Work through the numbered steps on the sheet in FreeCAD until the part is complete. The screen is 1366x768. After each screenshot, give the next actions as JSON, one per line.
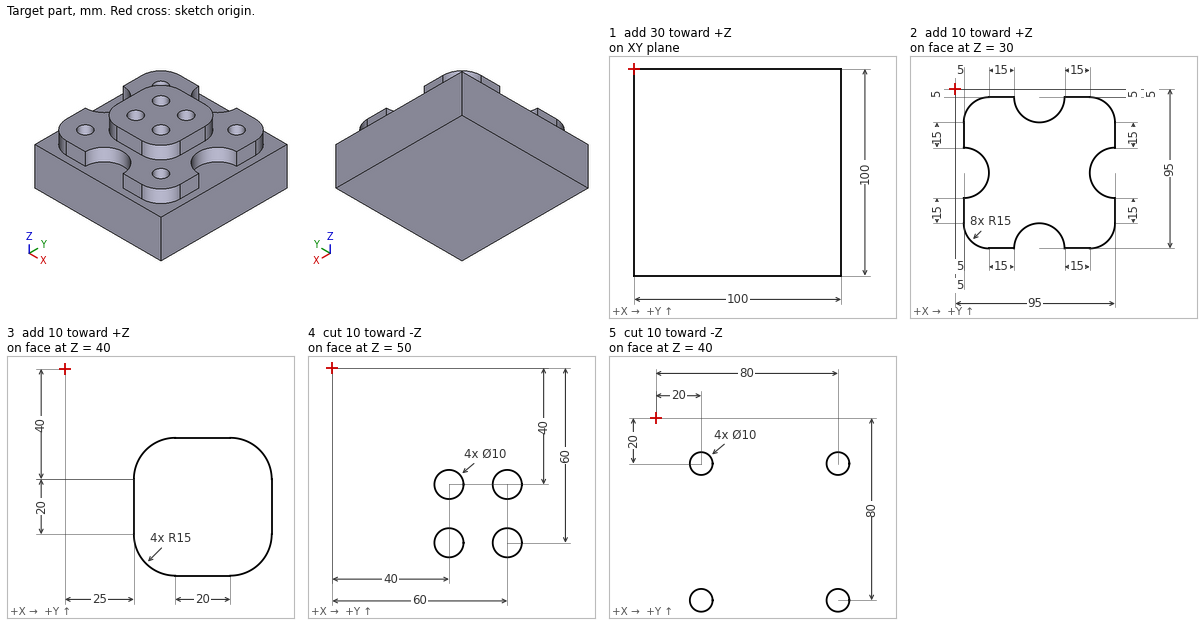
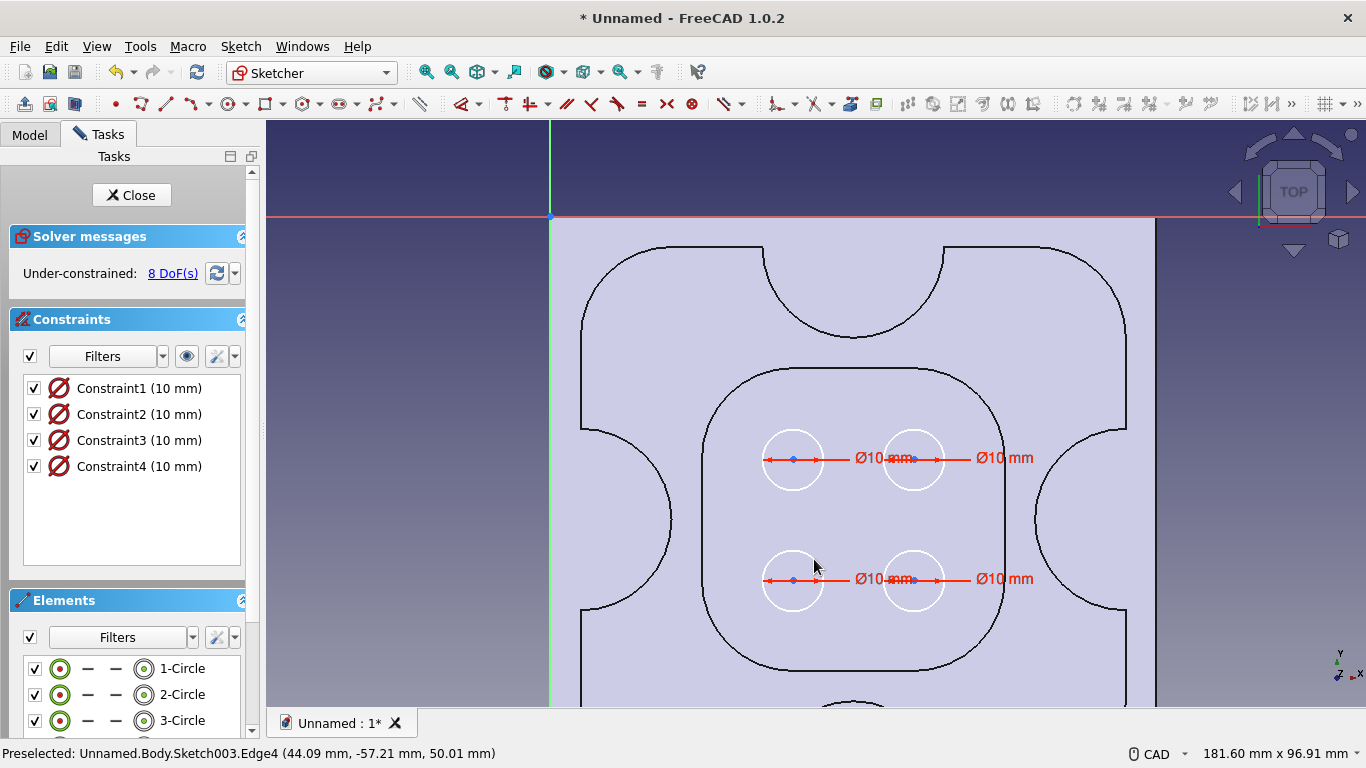
{"action": "left_click", "coordinate": [793, 460]}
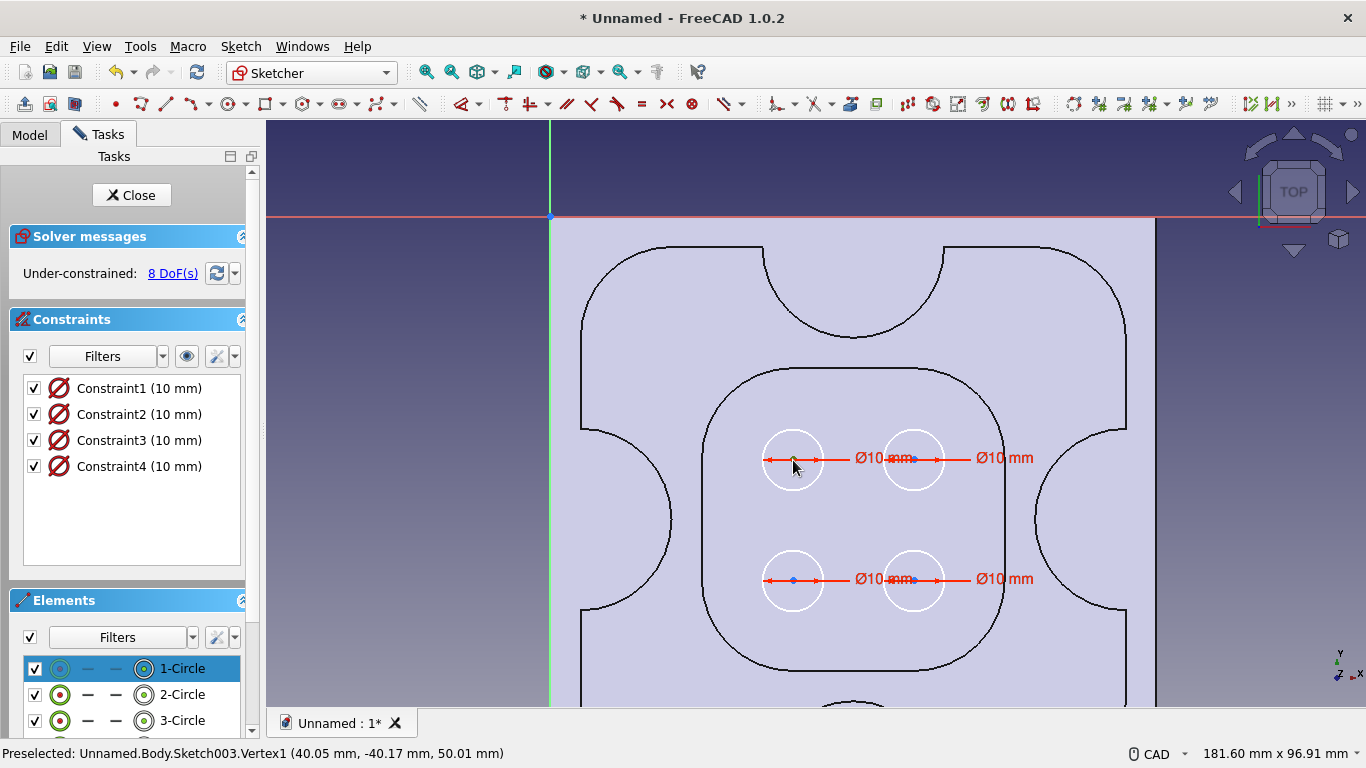
{"action": "left_click", "coordinate": [914, 460]}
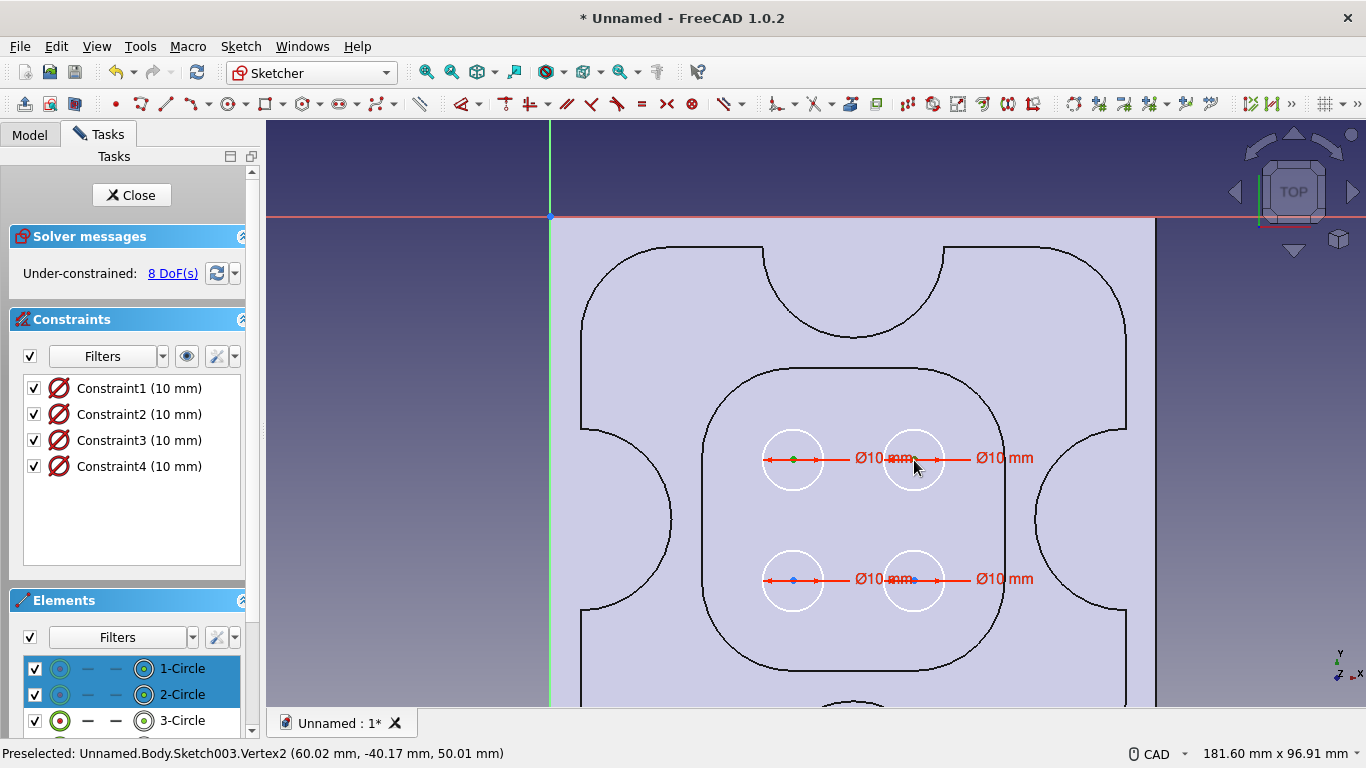
{"action": "left_click", "coordinate": [548, 104]}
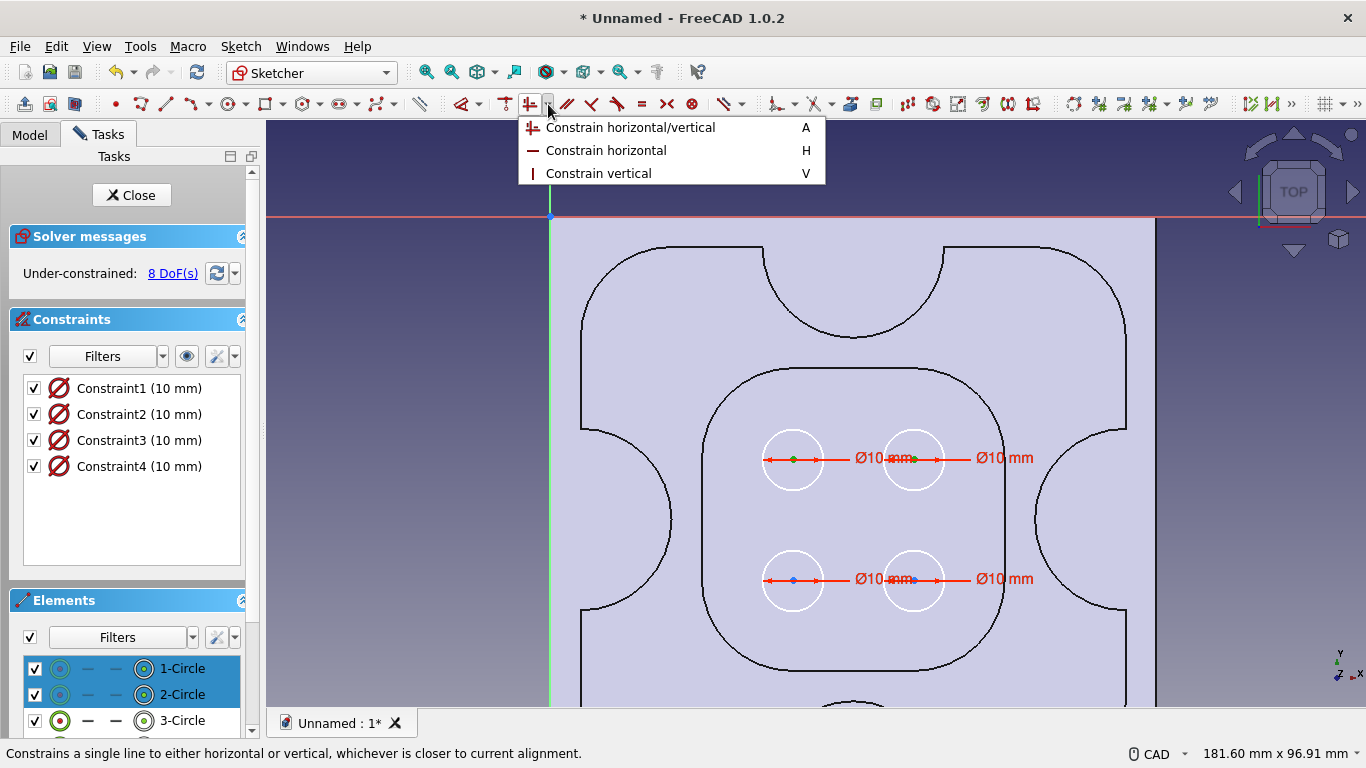
{"action": "left_click", "coordinate": [672, 150]}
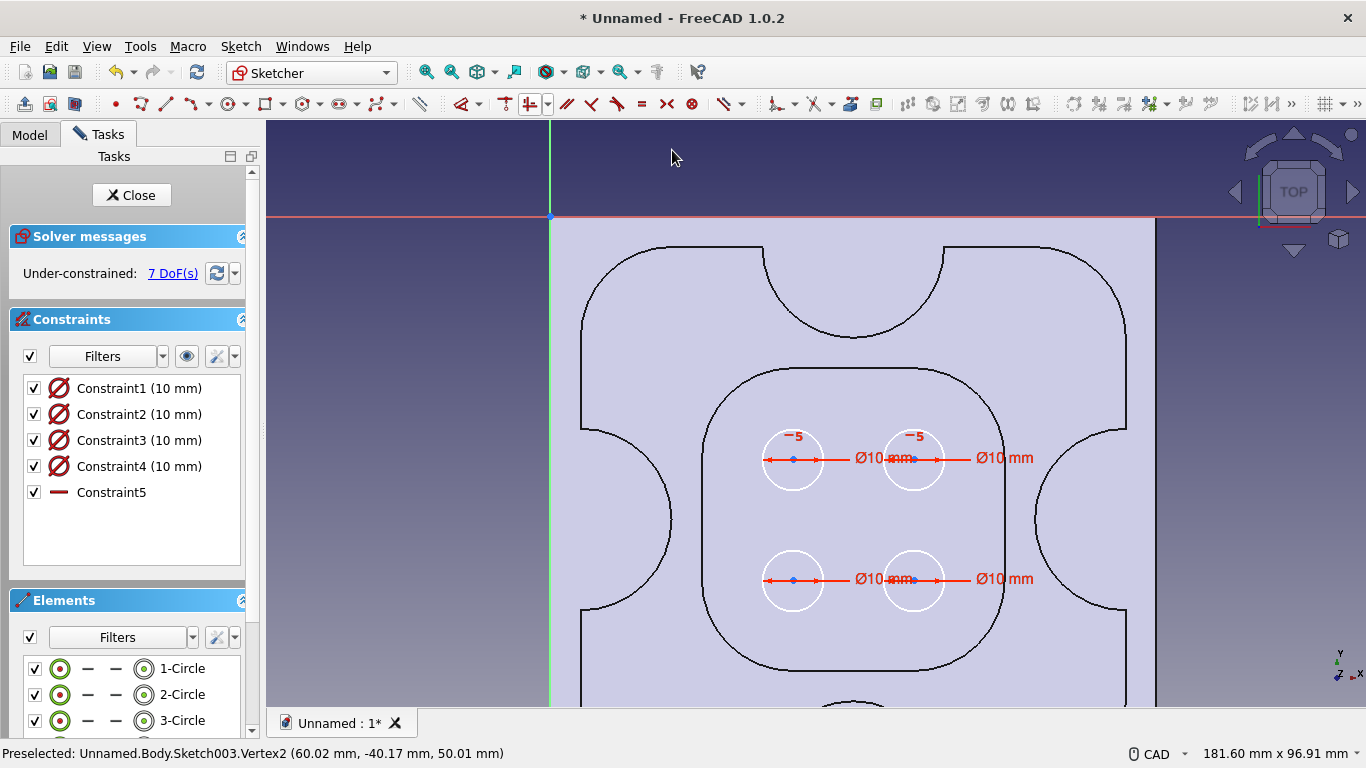
{"action": "left_click", "coordinate": [914, 460]}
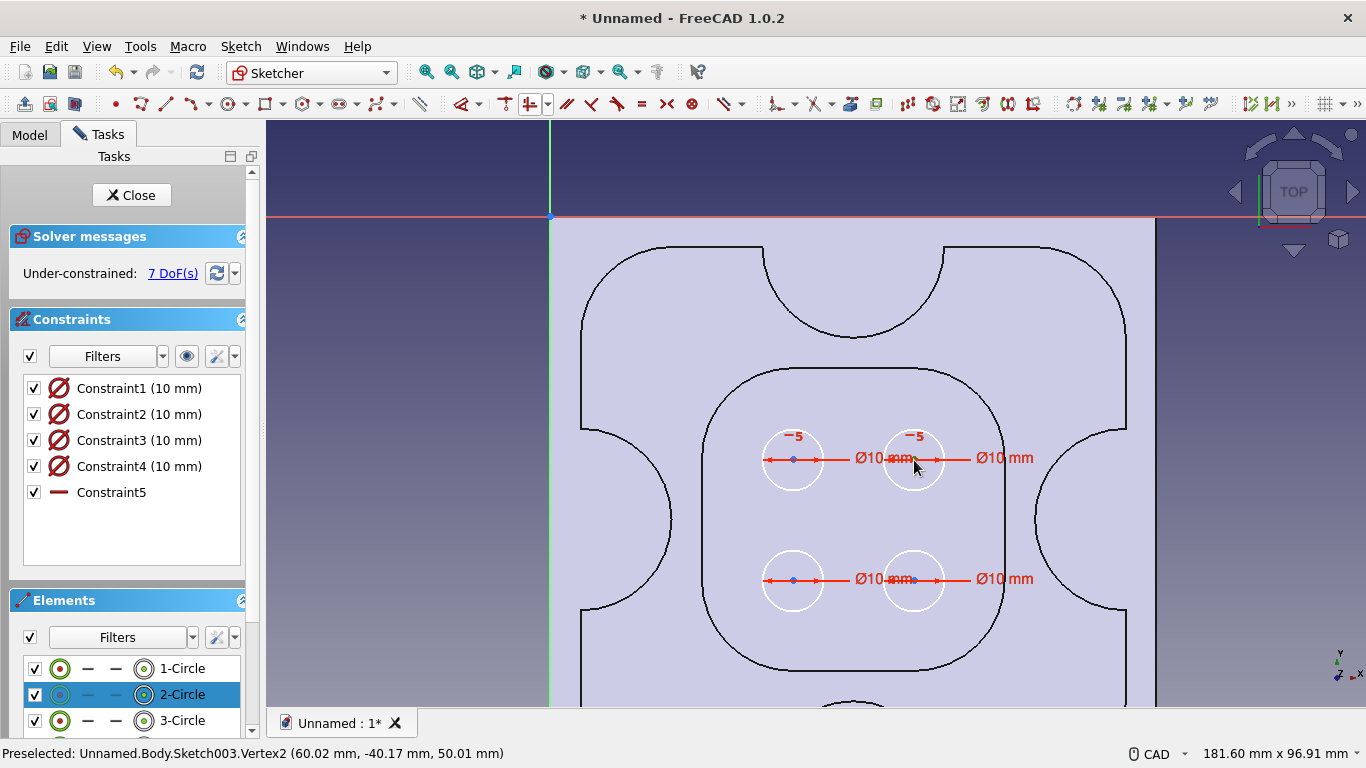
{"action": "left_click", "coordinate": [914, 581]}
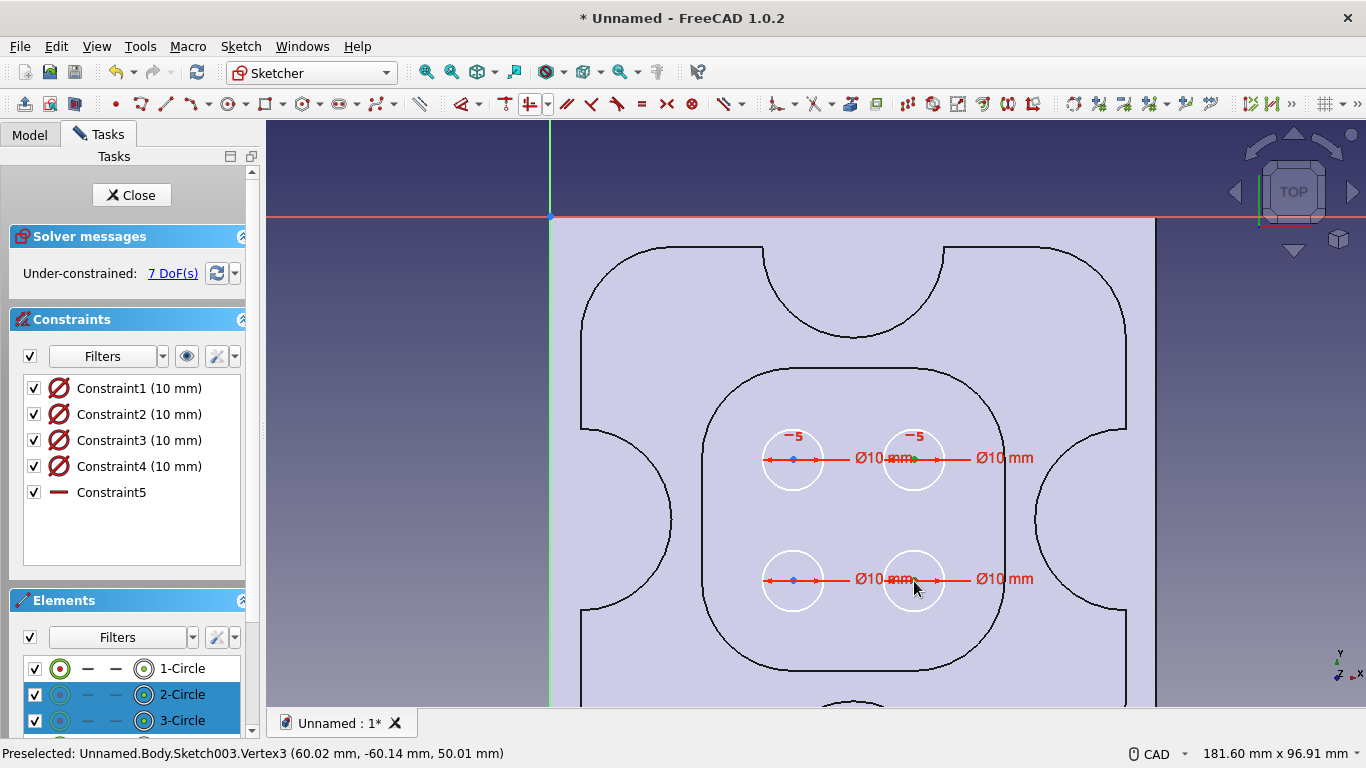
{"action": "key", "text": "v"}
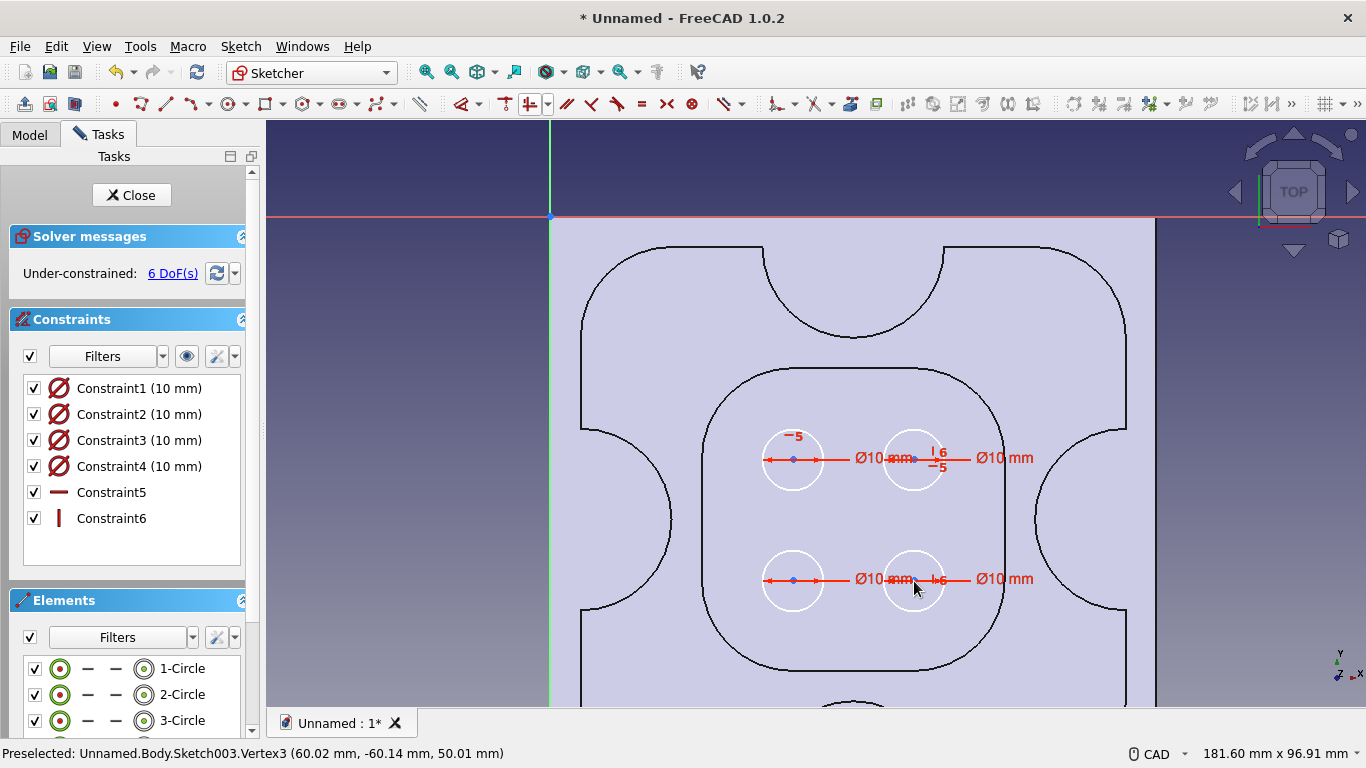
{"action": "left_click", "coordinate": [793, 460]}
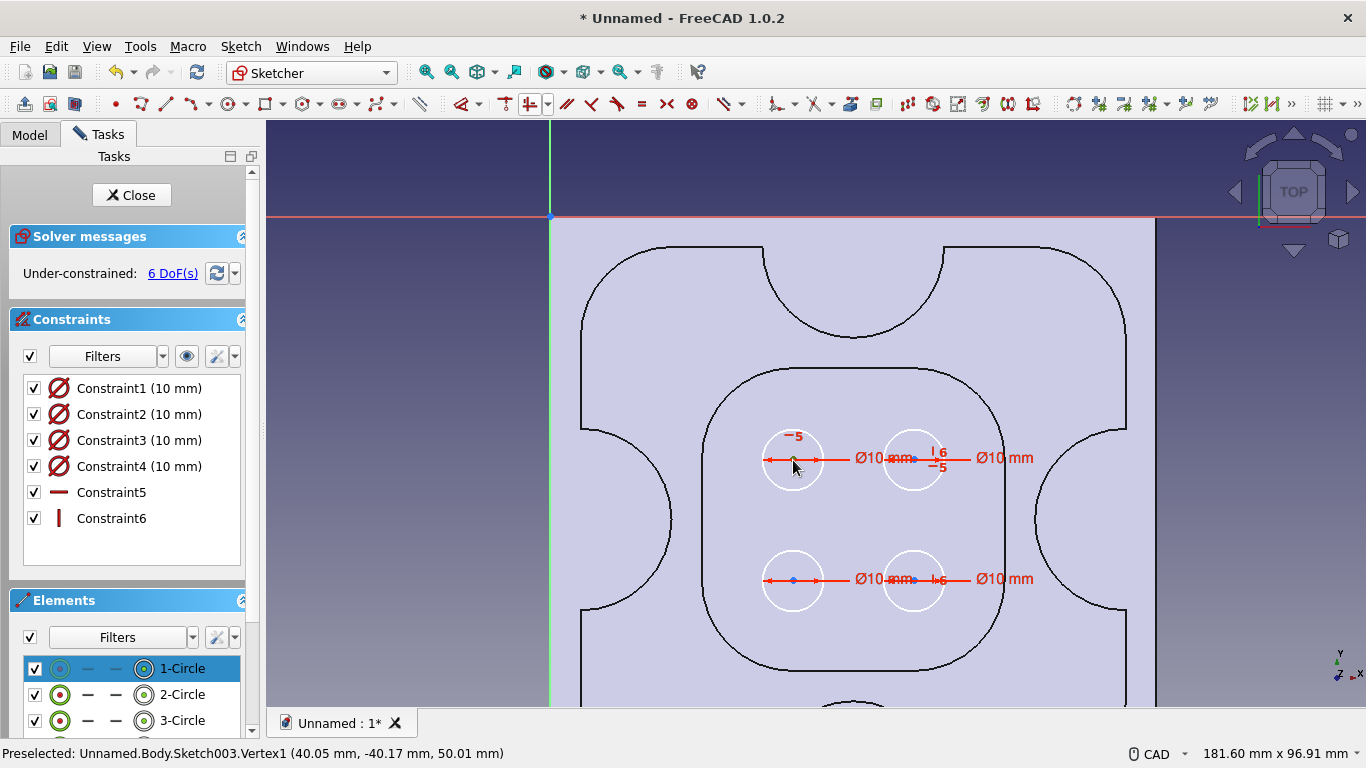
{"action": "left_click", "coordinate": [793, 581]}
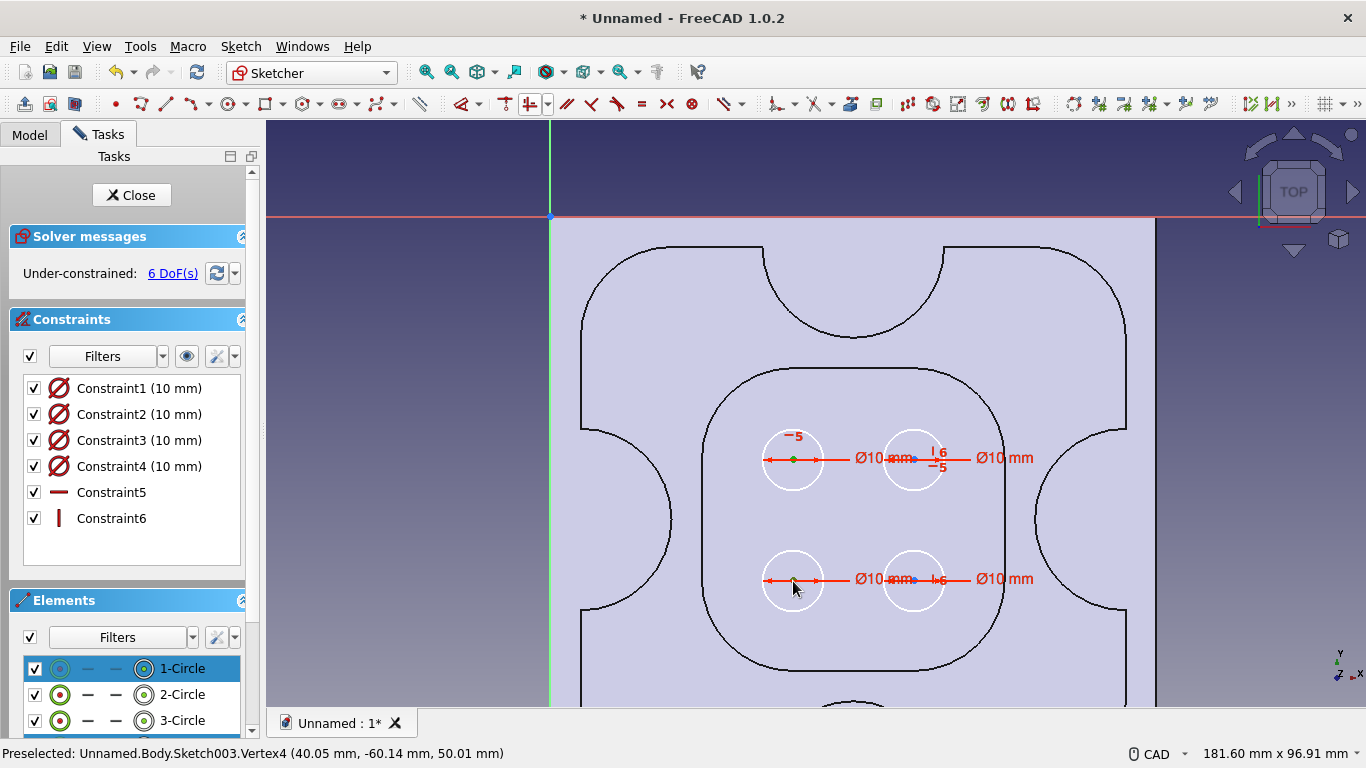
{"action": "left_click", "coordinate": [548, 104]}